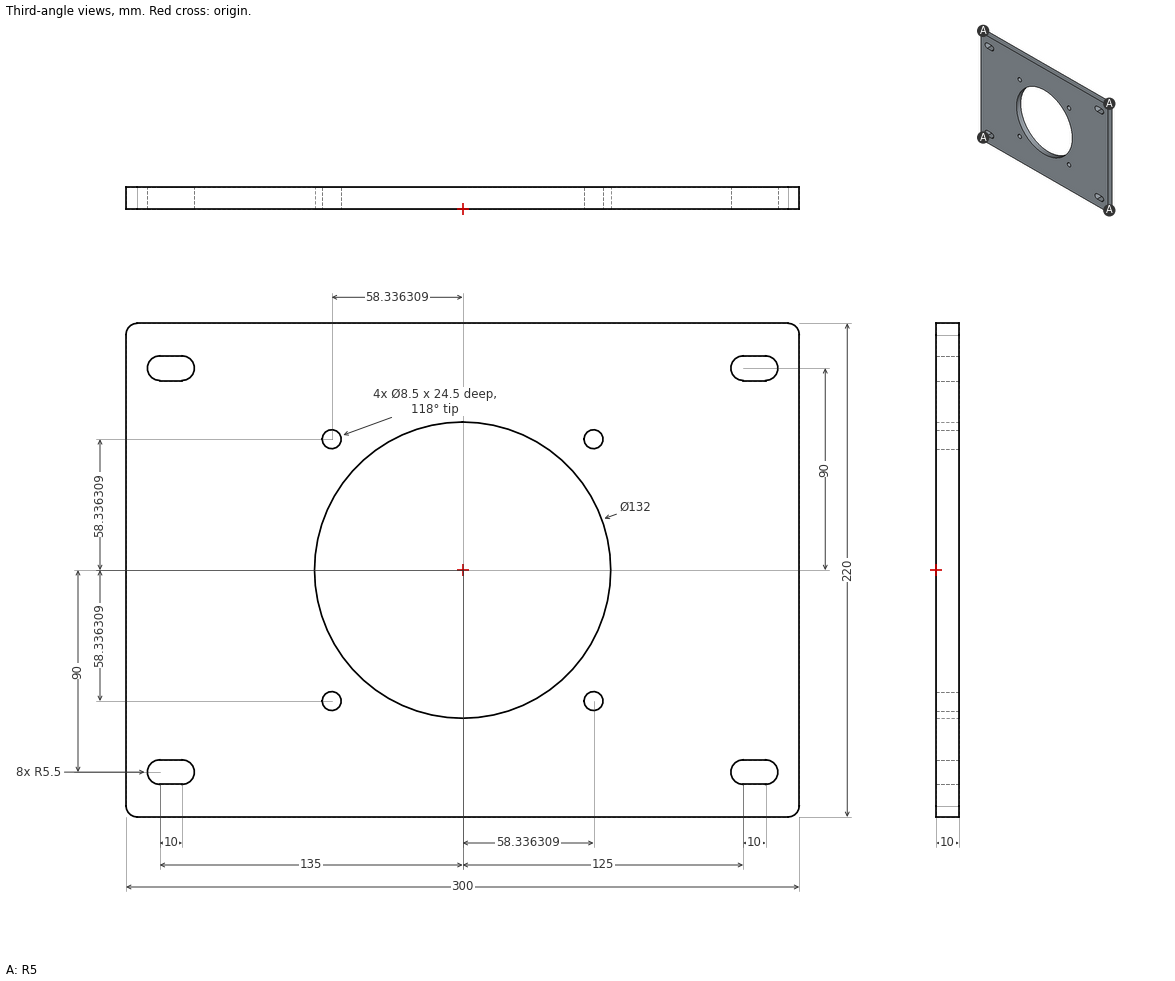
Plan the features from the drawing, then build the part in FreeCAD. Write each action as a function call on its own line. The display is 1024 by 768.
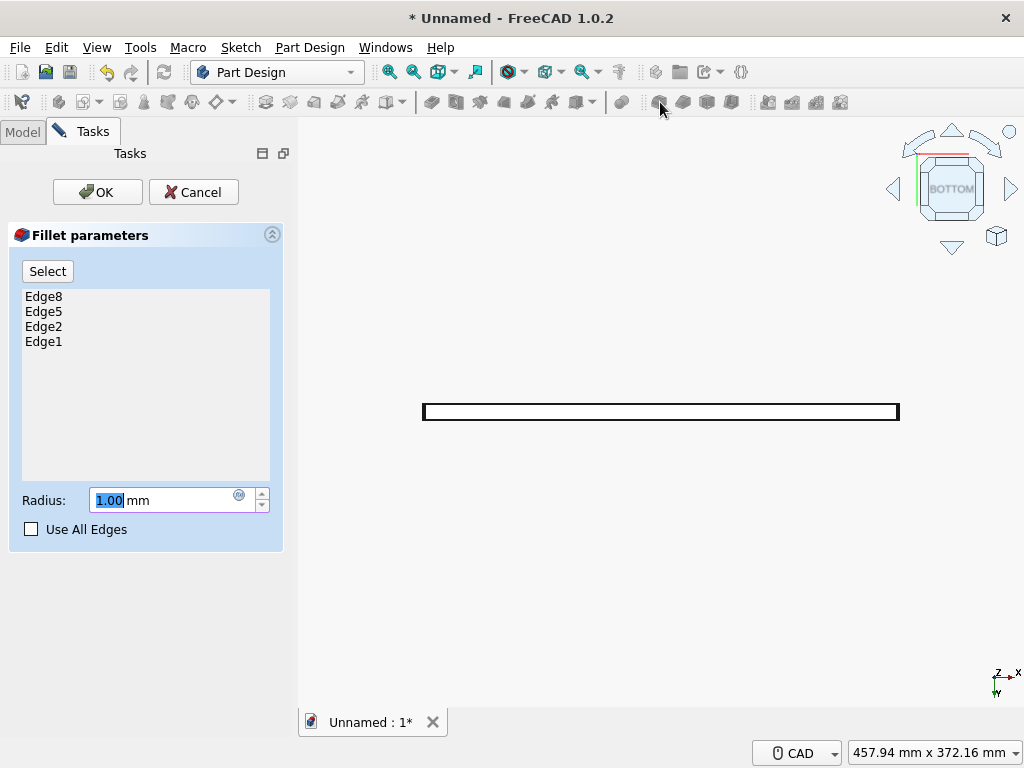
text(5)
key(Tab)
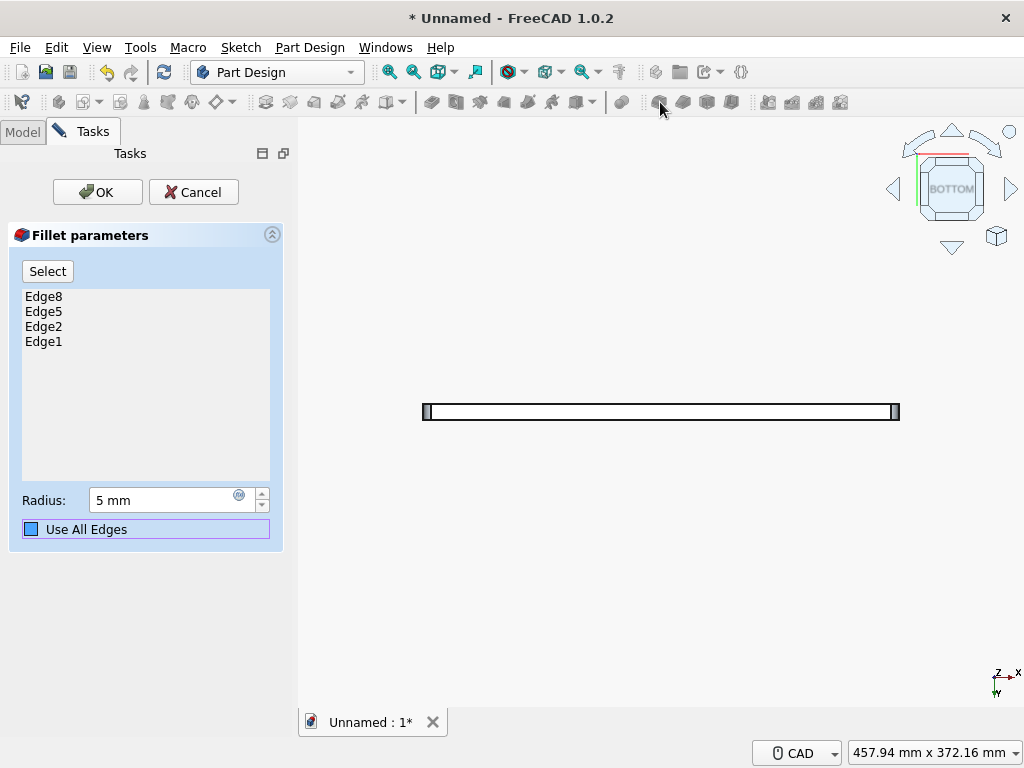
click(98, 192)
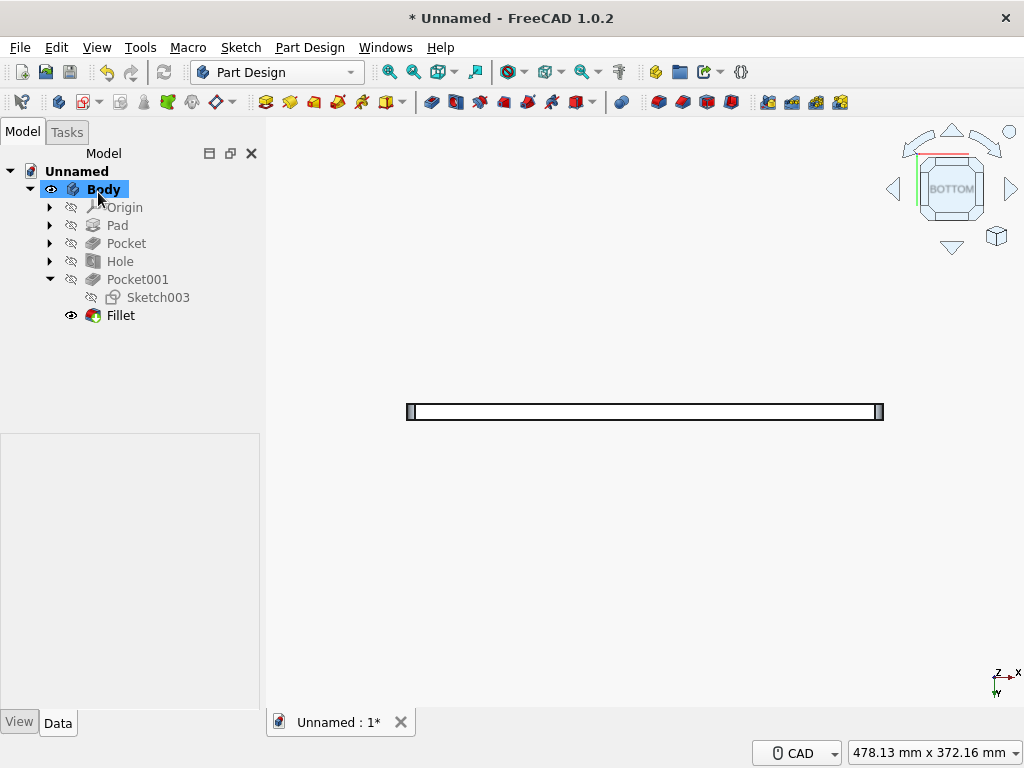
key(0)